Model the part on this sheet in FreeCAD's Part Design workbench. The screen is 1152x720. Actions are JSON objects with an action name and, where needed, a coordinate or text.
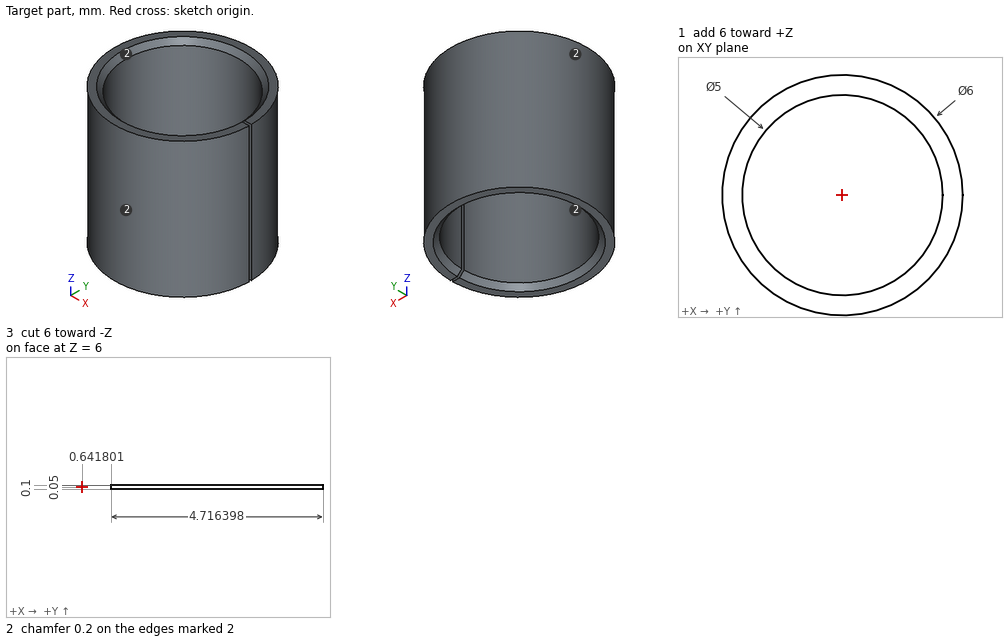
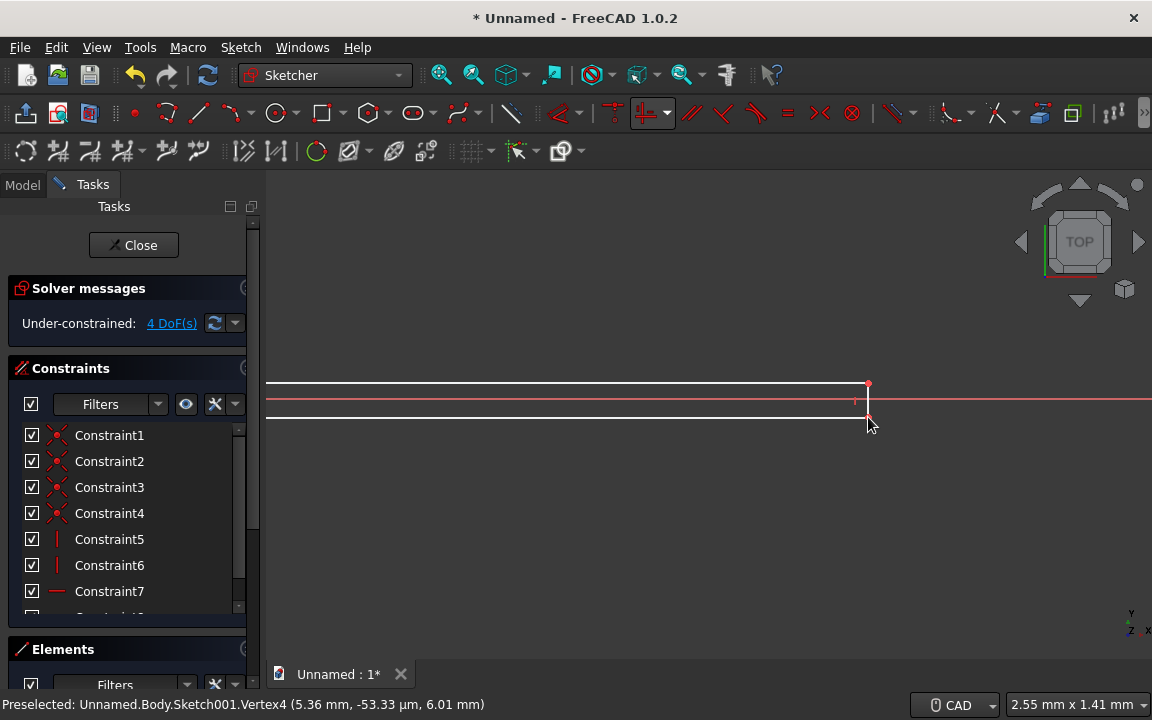
{"action": "left_click", "coordinate": [558, 114]}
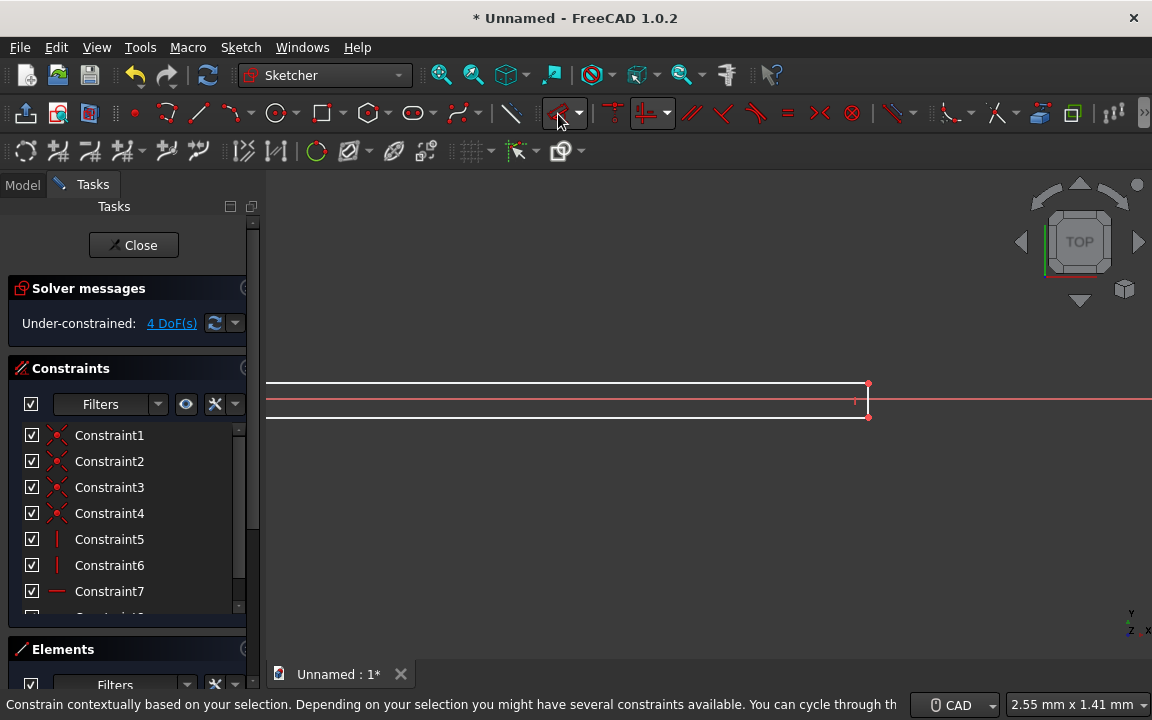
{"action": "scroll", "coordinate": [871, 419], "scroll_direction": "down", "scroll_amount": 7}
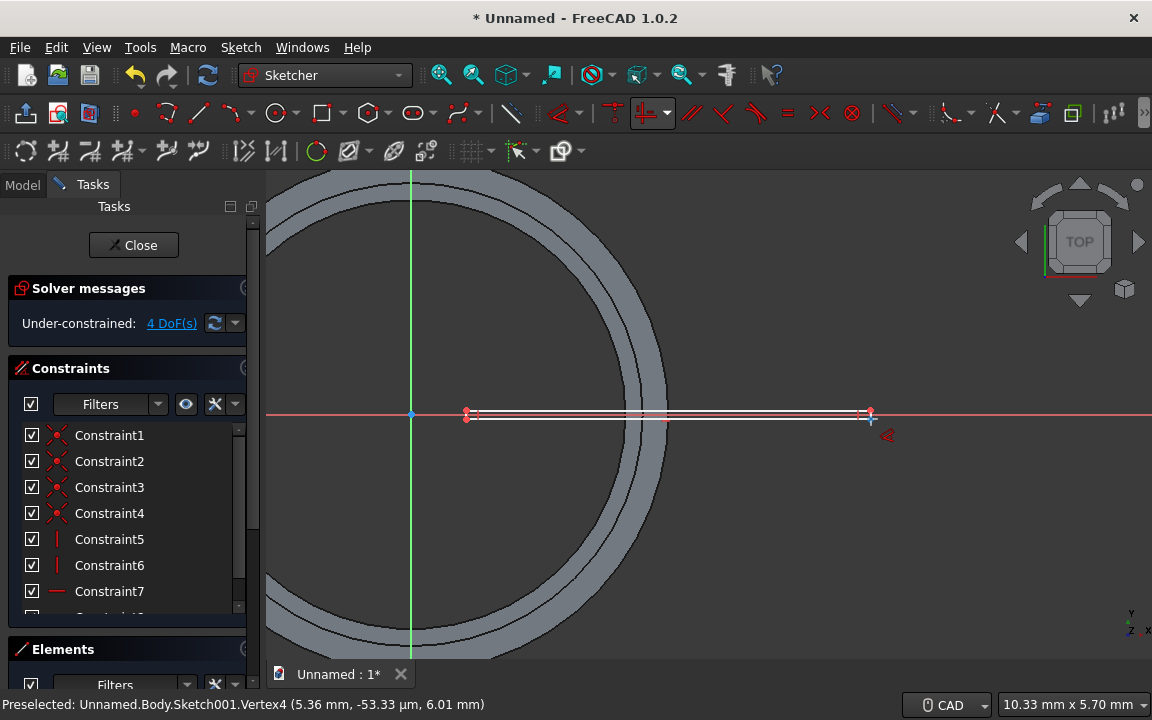
{"action": "scroll", "coordinate": [466, 414], "scroll_direction": "up", "scroll_amount": 8}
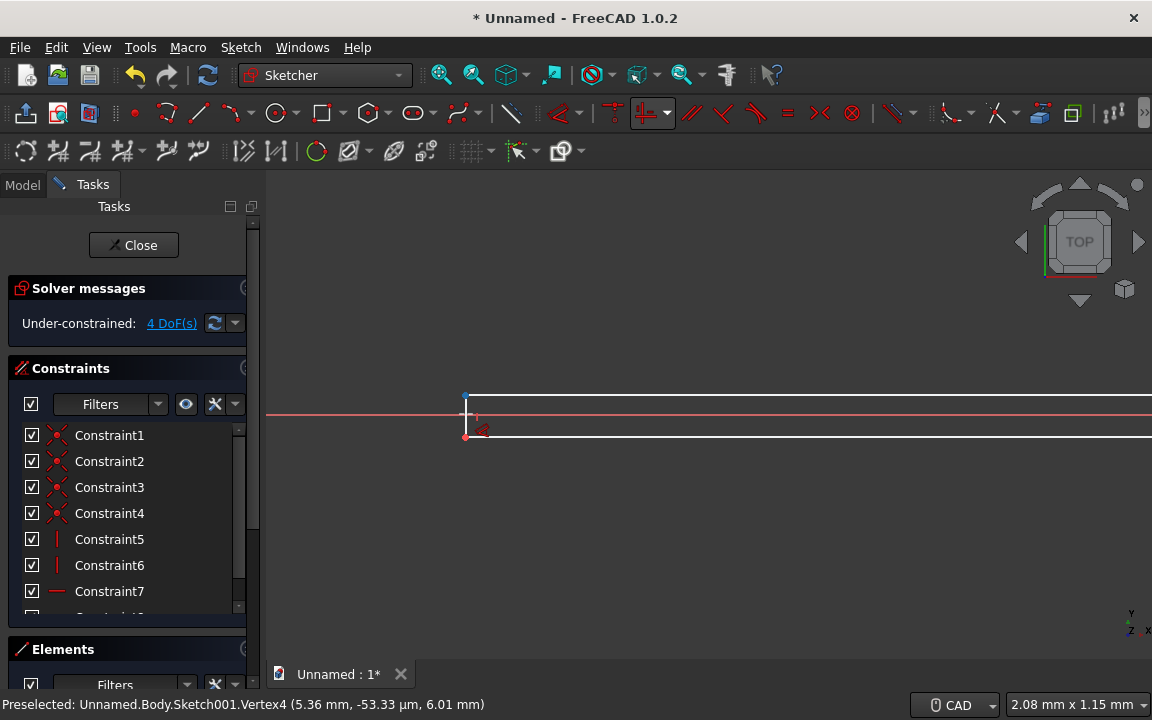
{"action": "left_click", "coordinate": [466, 412]}
{"action": "left_click", "coordinate": [432, 402]}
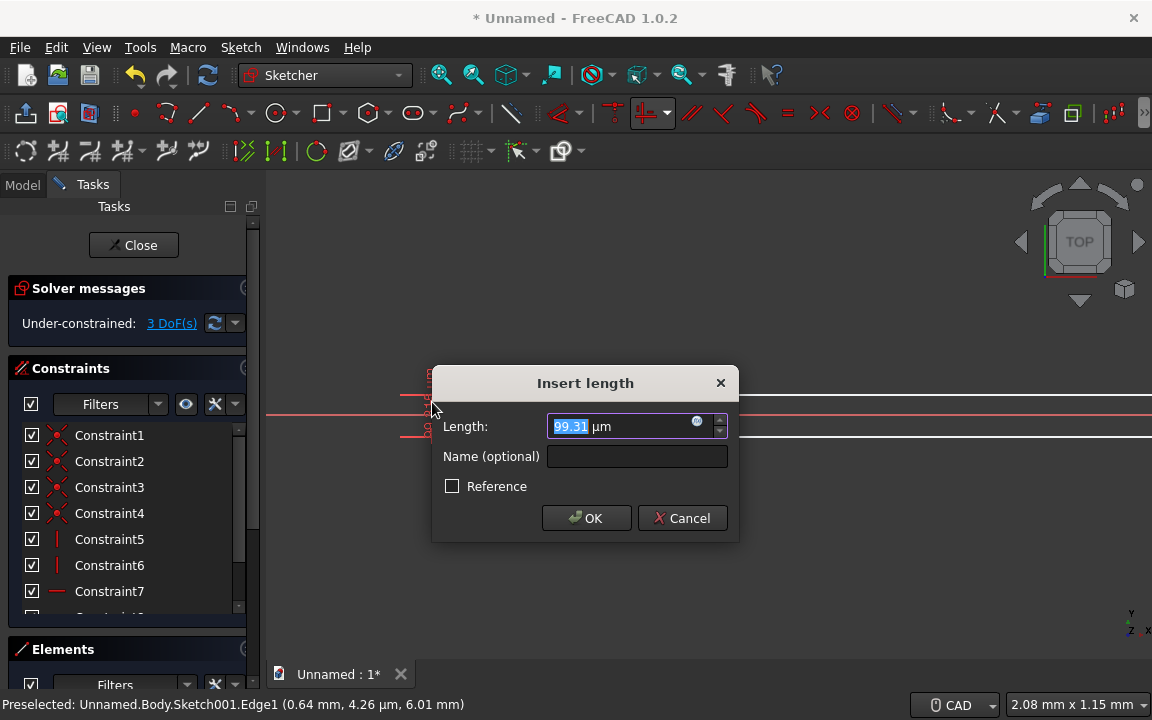
{"action": "key", "text": "ctrl+a"}
{"action": "type", "text": "0.1 mm"}
{"action": "key", "text": "Return"}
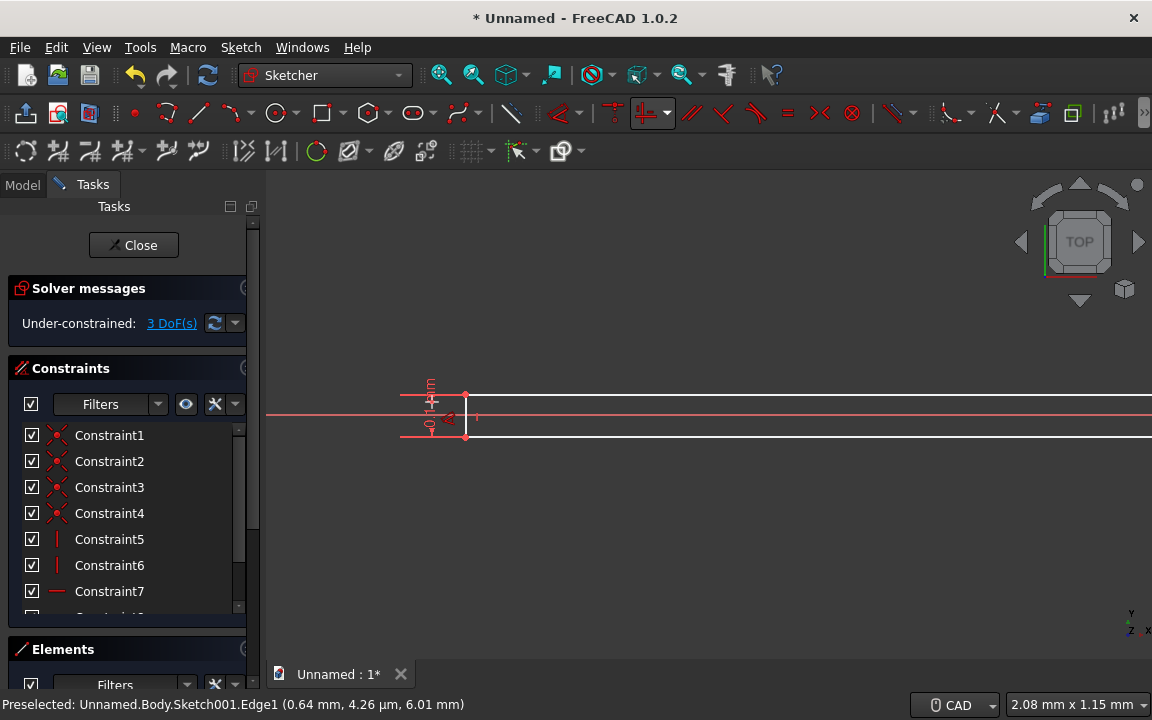
{"action": "scroll", "coordinate": [466, 395], "scroll_direction": "up", "scroll_amount": 4}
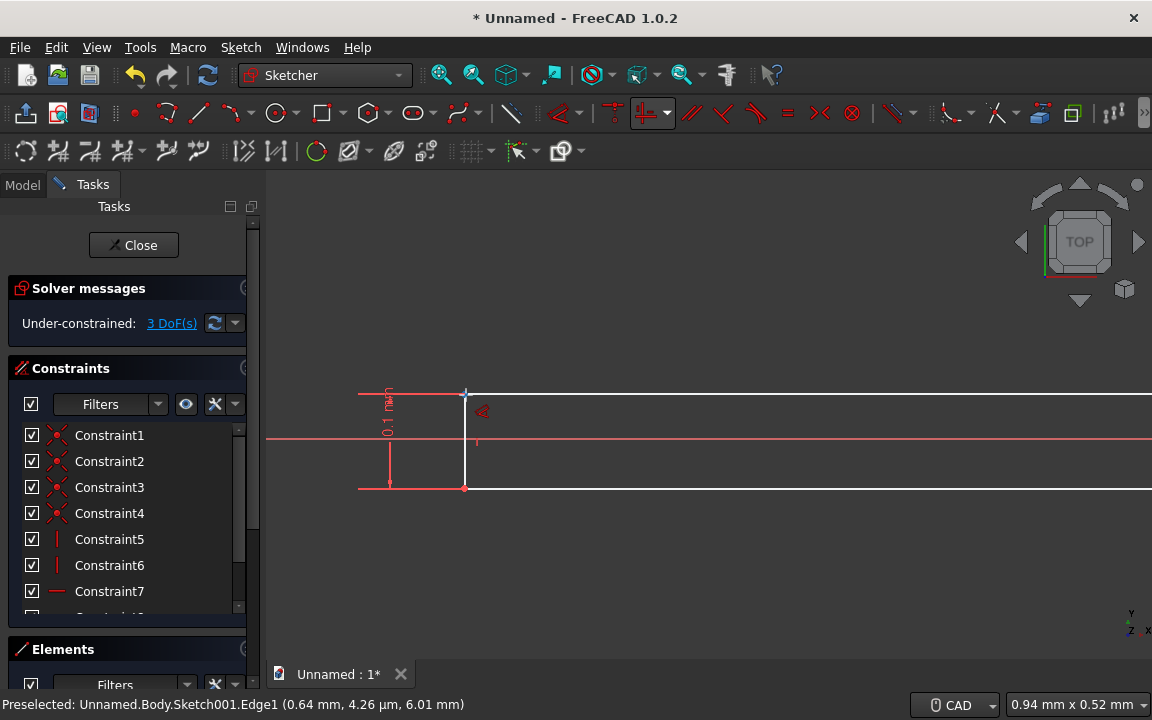
{"action": "left_click", "coordinate": [465, 394]}
{"action": "left_click", "coordinate": [499, 416]}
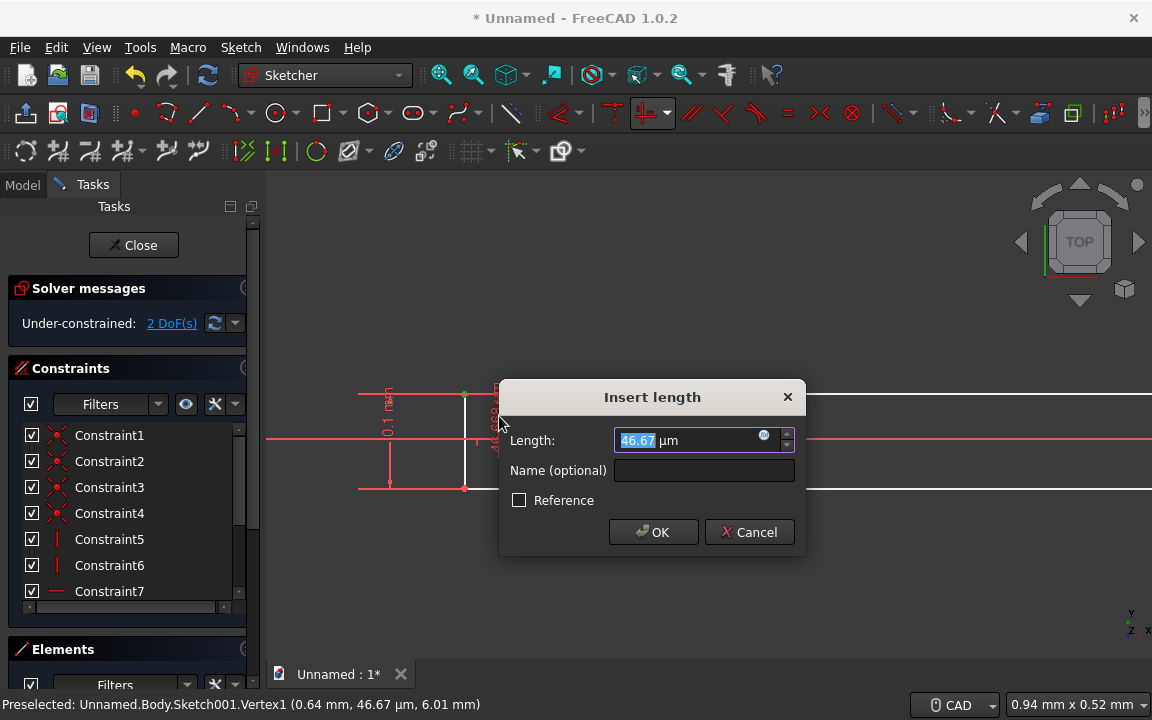
{"action": "key", "text": "ctrl+a"}
{"action": "type", "text": "0.05 mm"}
{"action": "key", "text": "Return"}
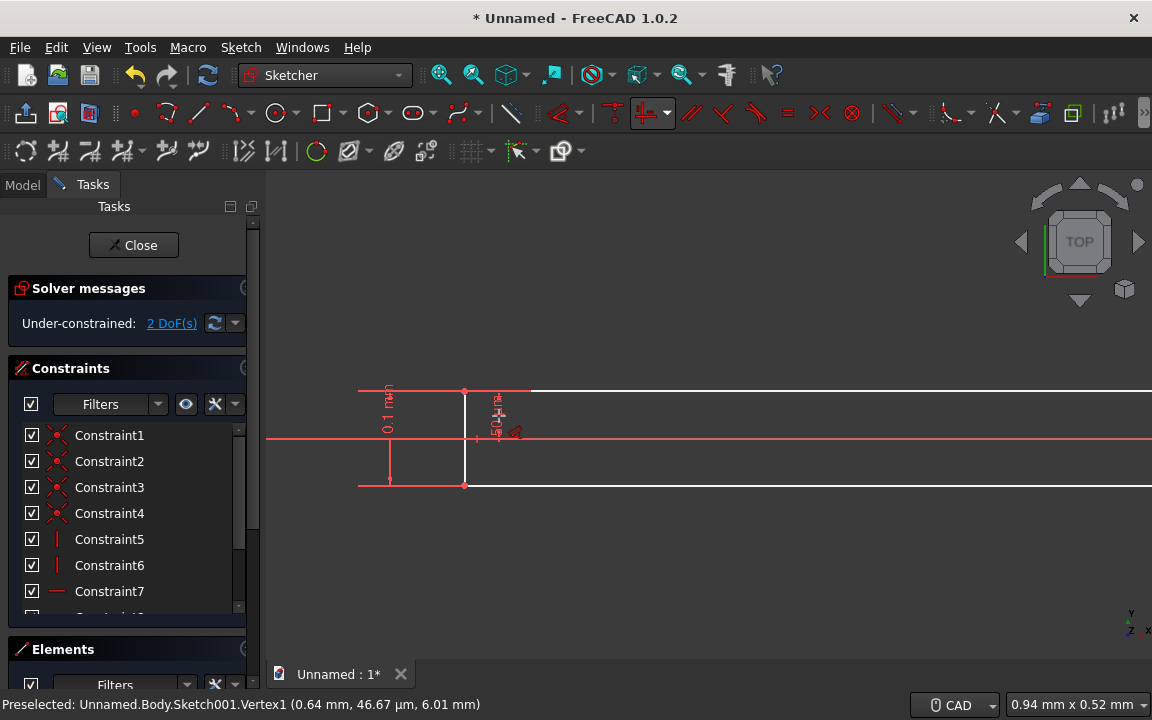
{"action": "scroll", "coordinate": [466, 412], "scroll_direction": "down", "scroll_amount": 12}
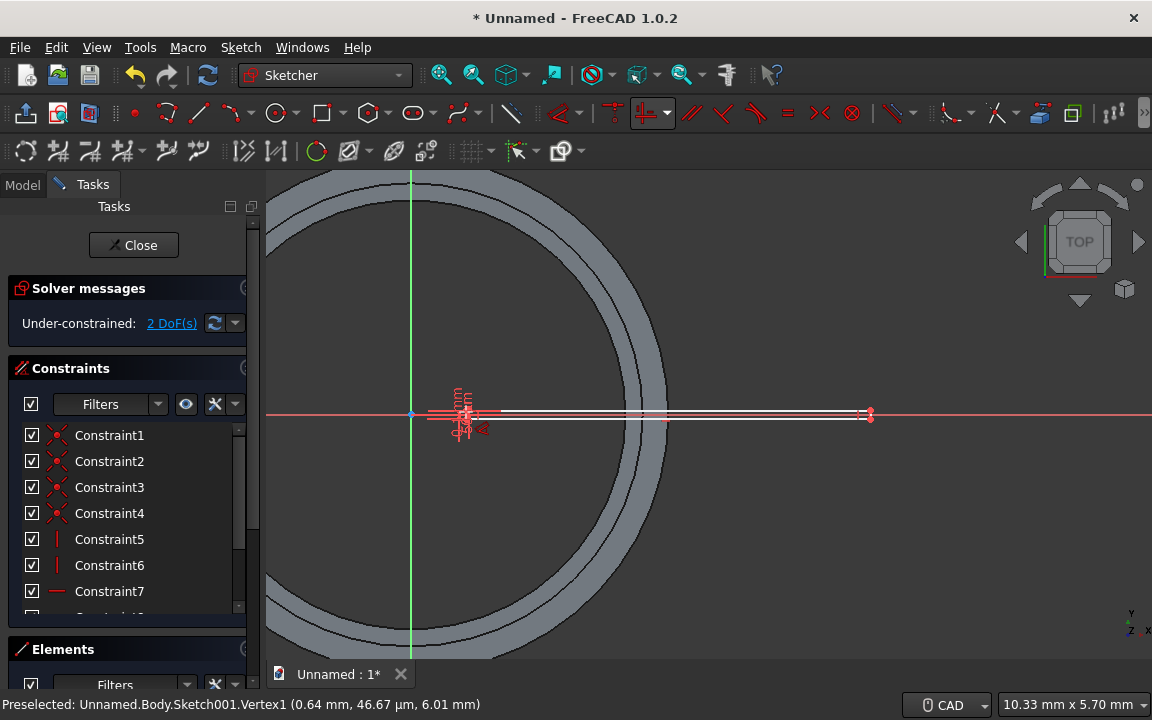
{"action": "scroll", "coordinate": [588, 419], "scroll_direction": "up", "scroll_amount": 6}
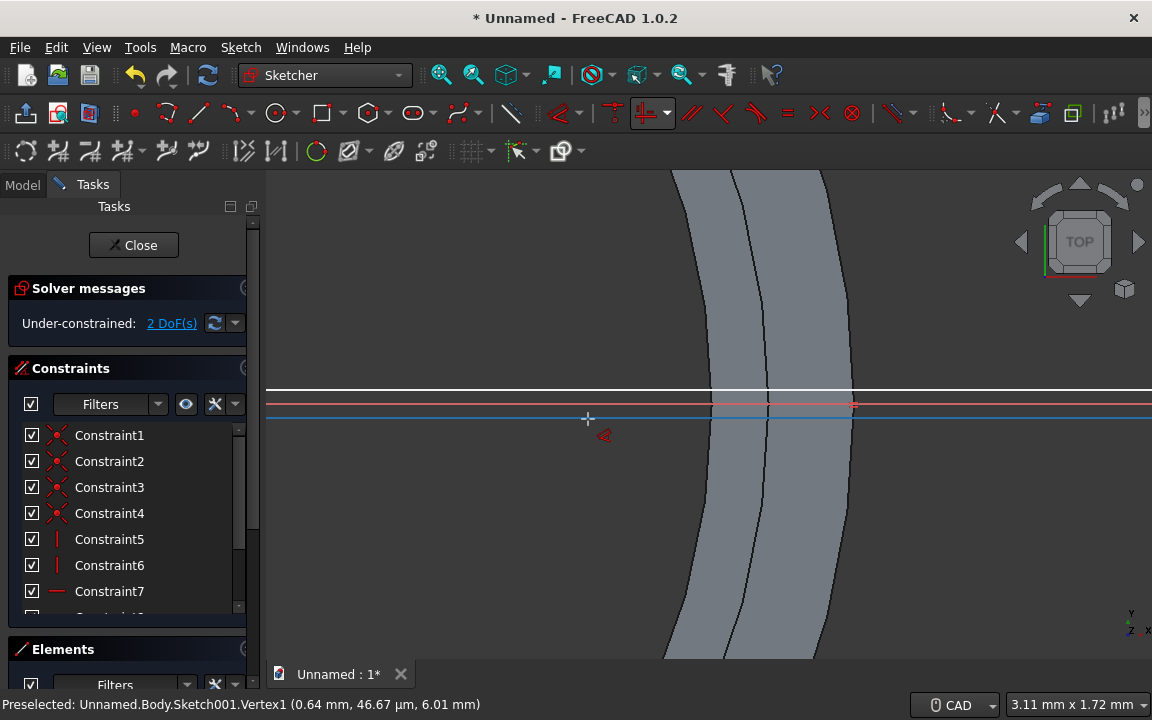
{"action": "left_click", "coordinate": [586, 418]}
{"action": "left_click", "coordinate": [640, 452]}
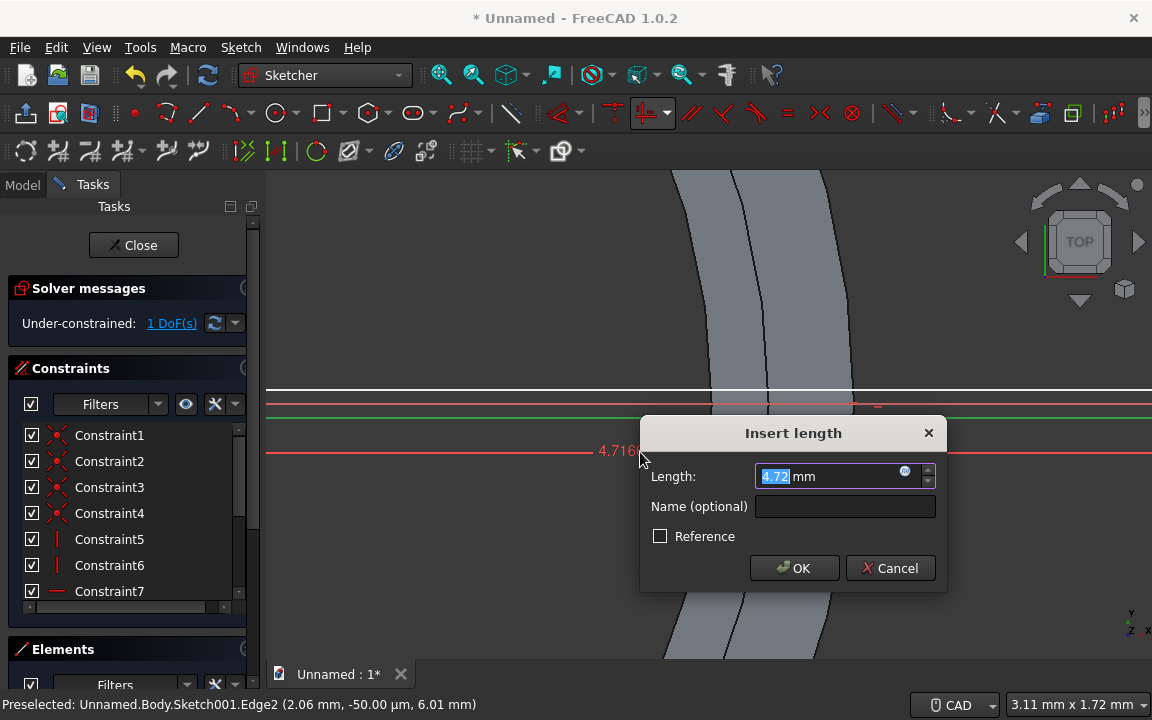
{"action": "type", "text": "4.716398"}
{"action": "key", "text": "Return"}